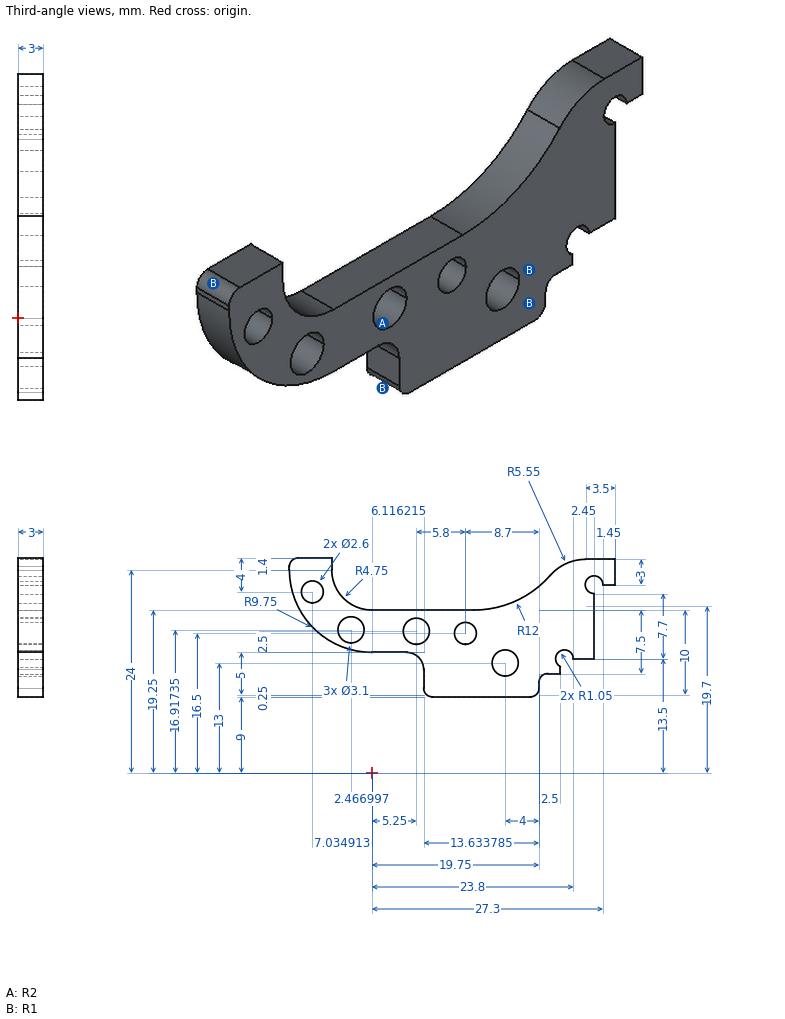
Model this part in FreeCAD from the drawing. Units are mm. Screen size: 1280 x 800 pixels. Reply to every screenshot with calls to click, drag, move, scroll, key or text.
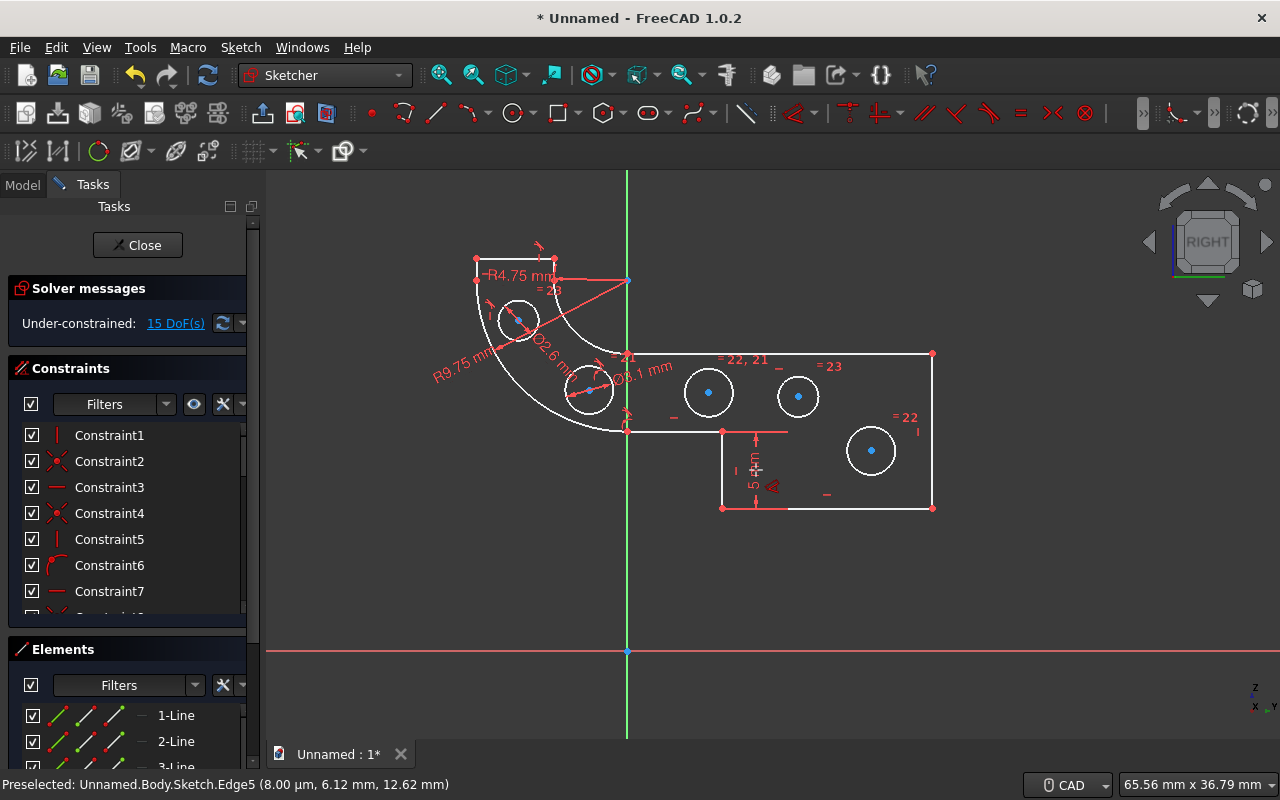
click(932, 462)
click(966, 431)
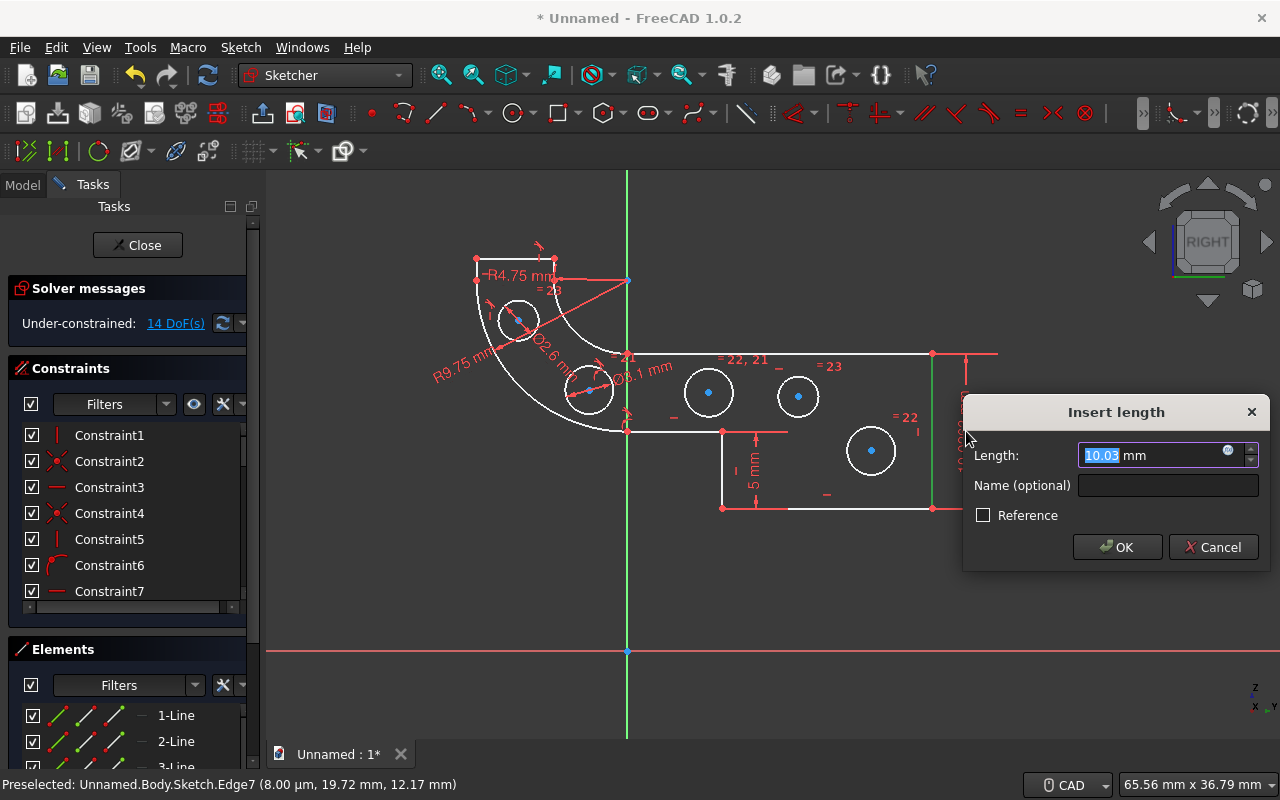
text(10)
key(Return)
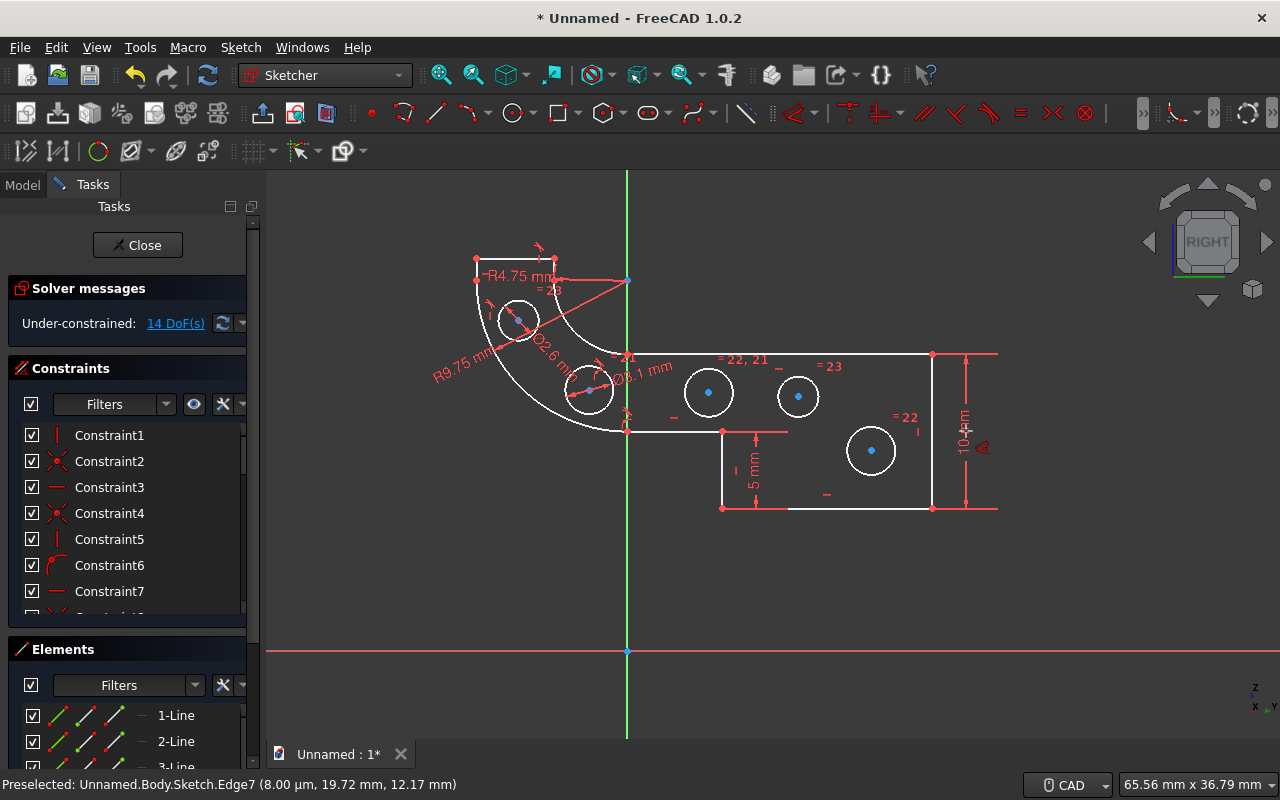
click(871, 451)
click(905, 551)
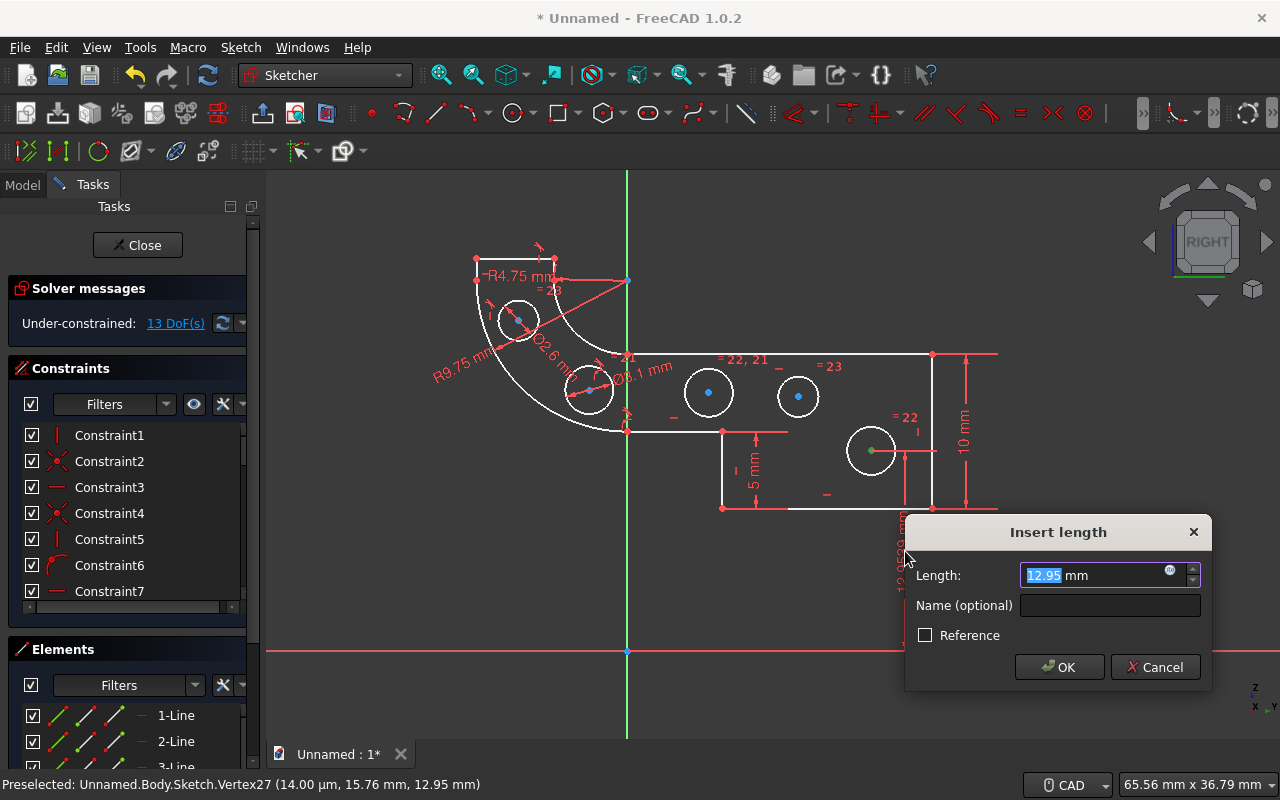
text(13)
key(Return)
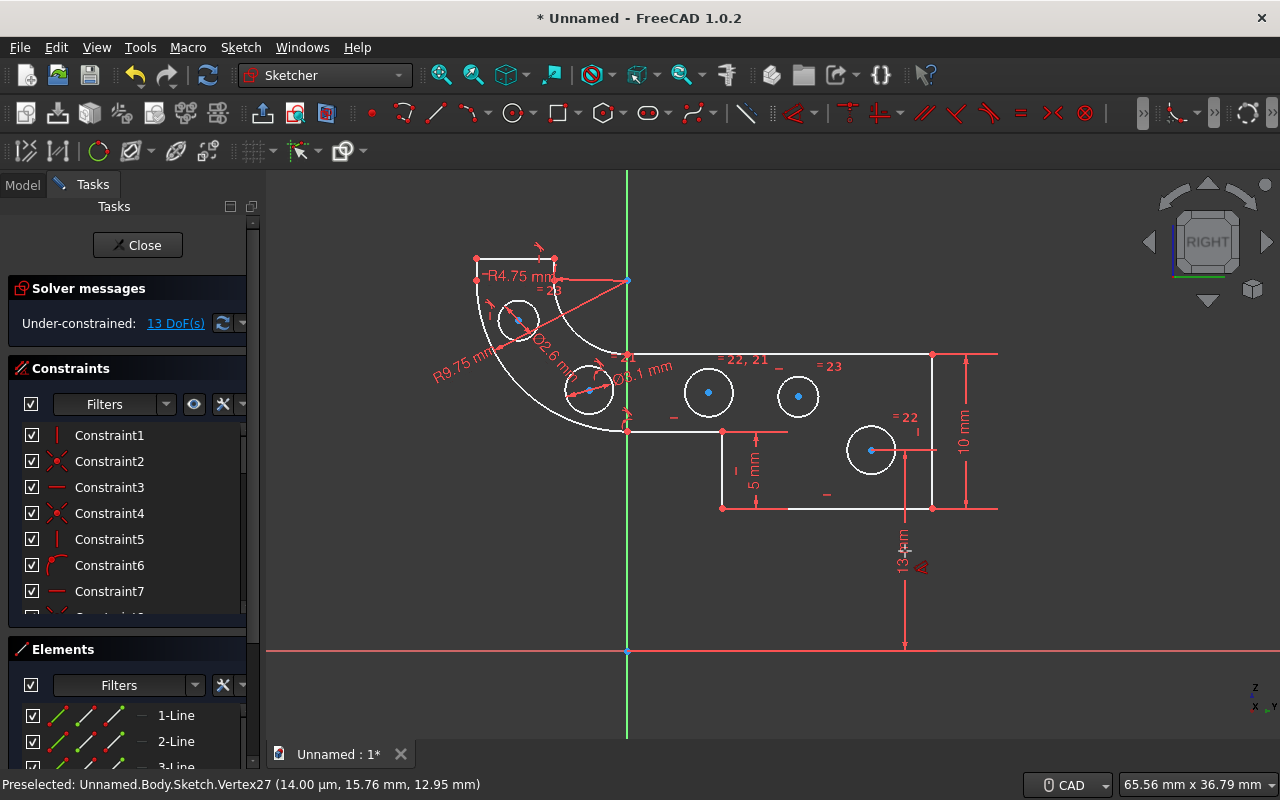
click(554, 259)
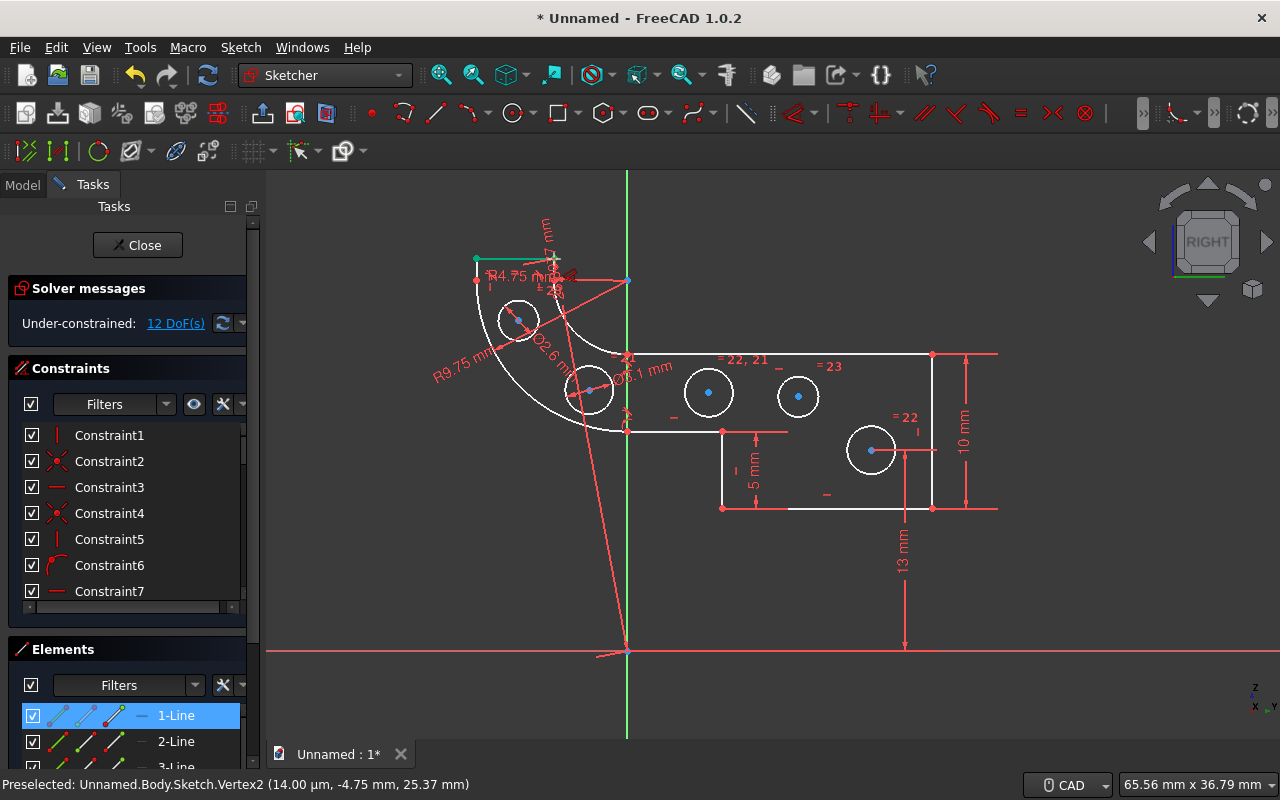
click(519, 321)
click(588, 304)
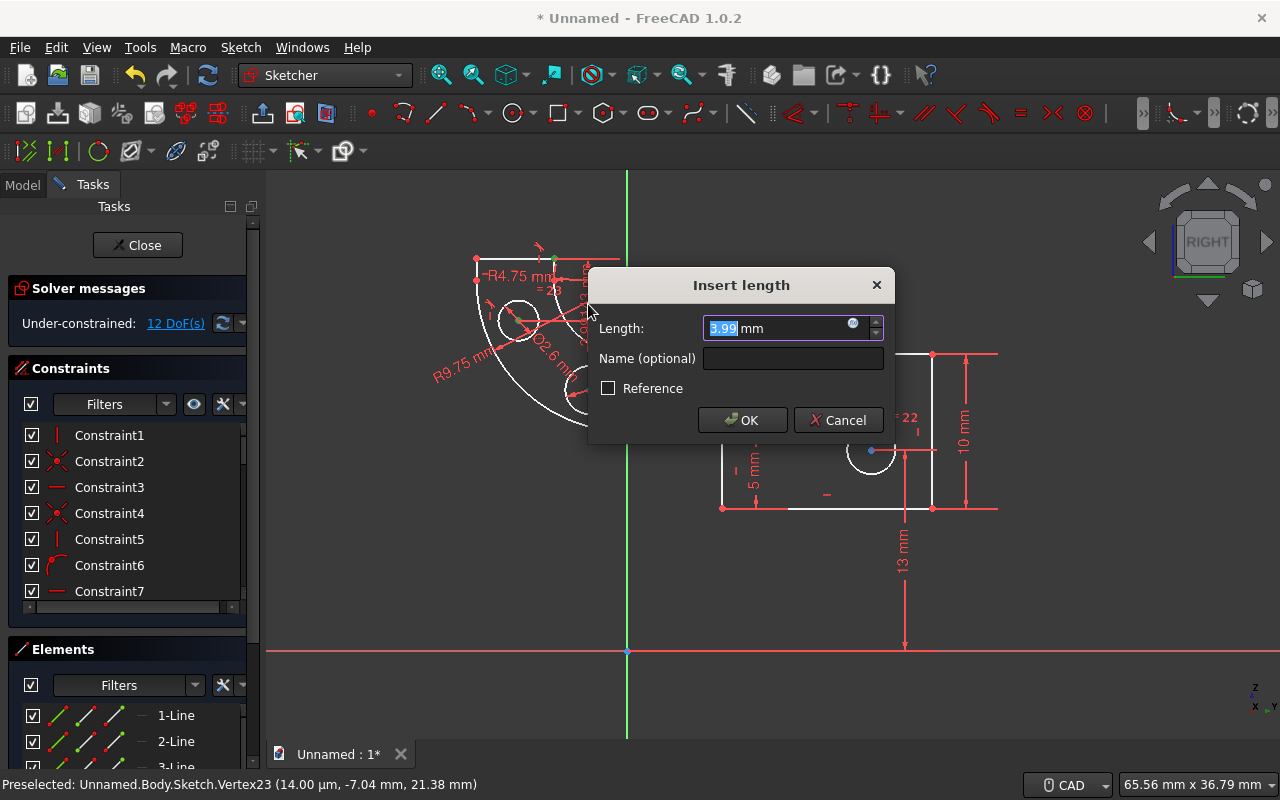
text(4)
key(Return)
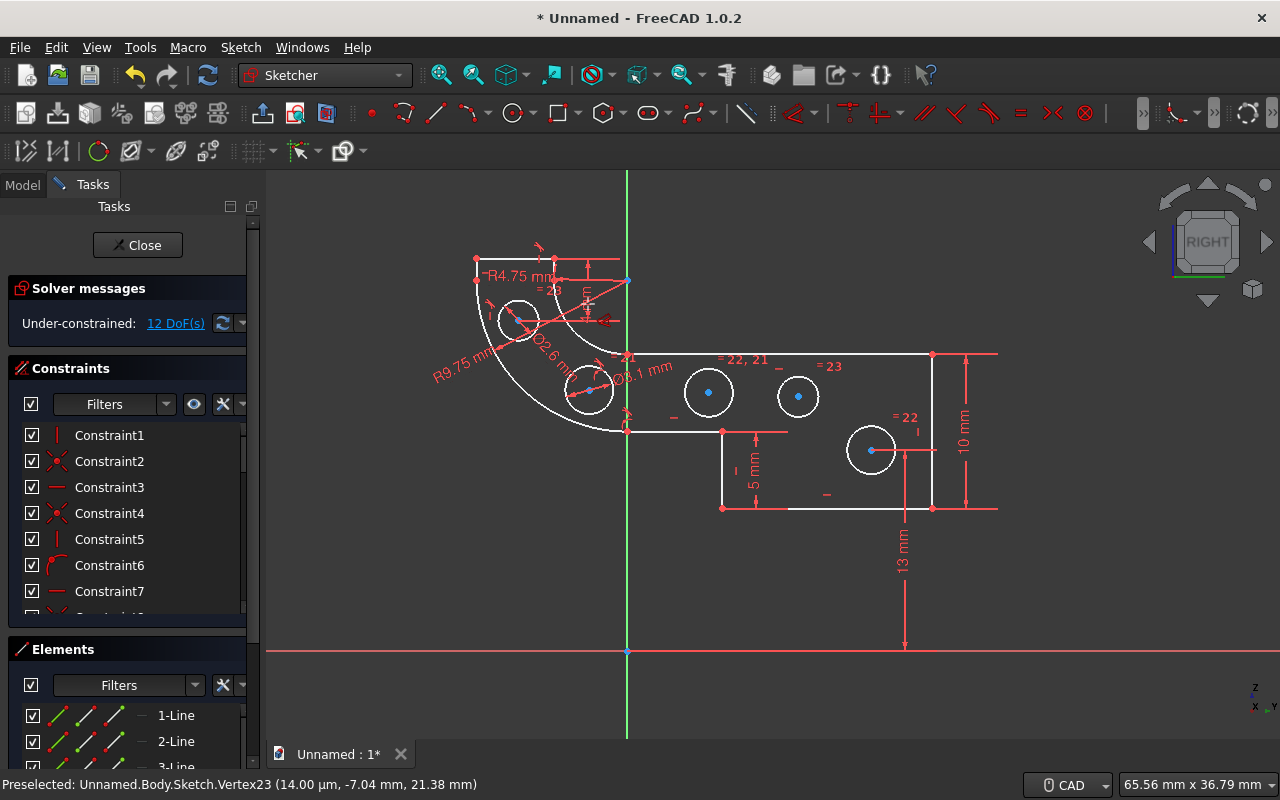
click(932, 509)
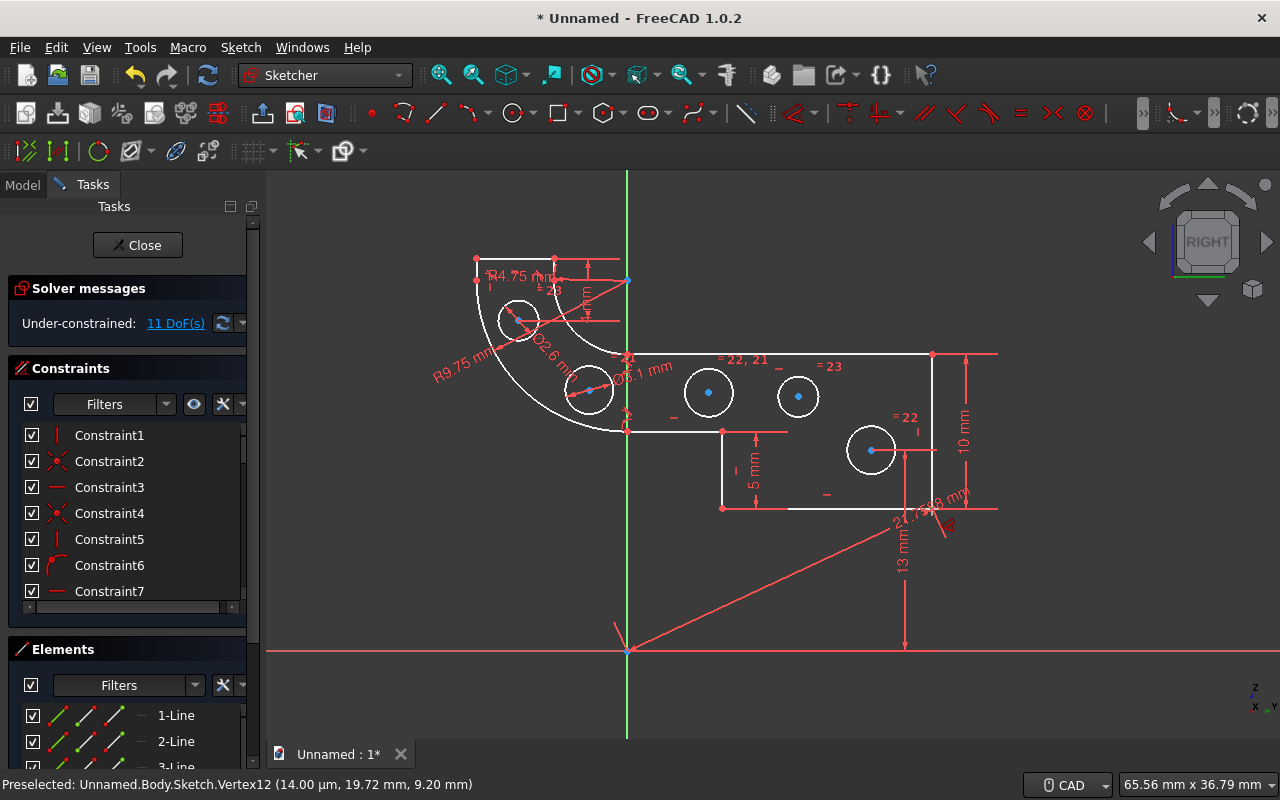
click(871, 450)
click(888, 416)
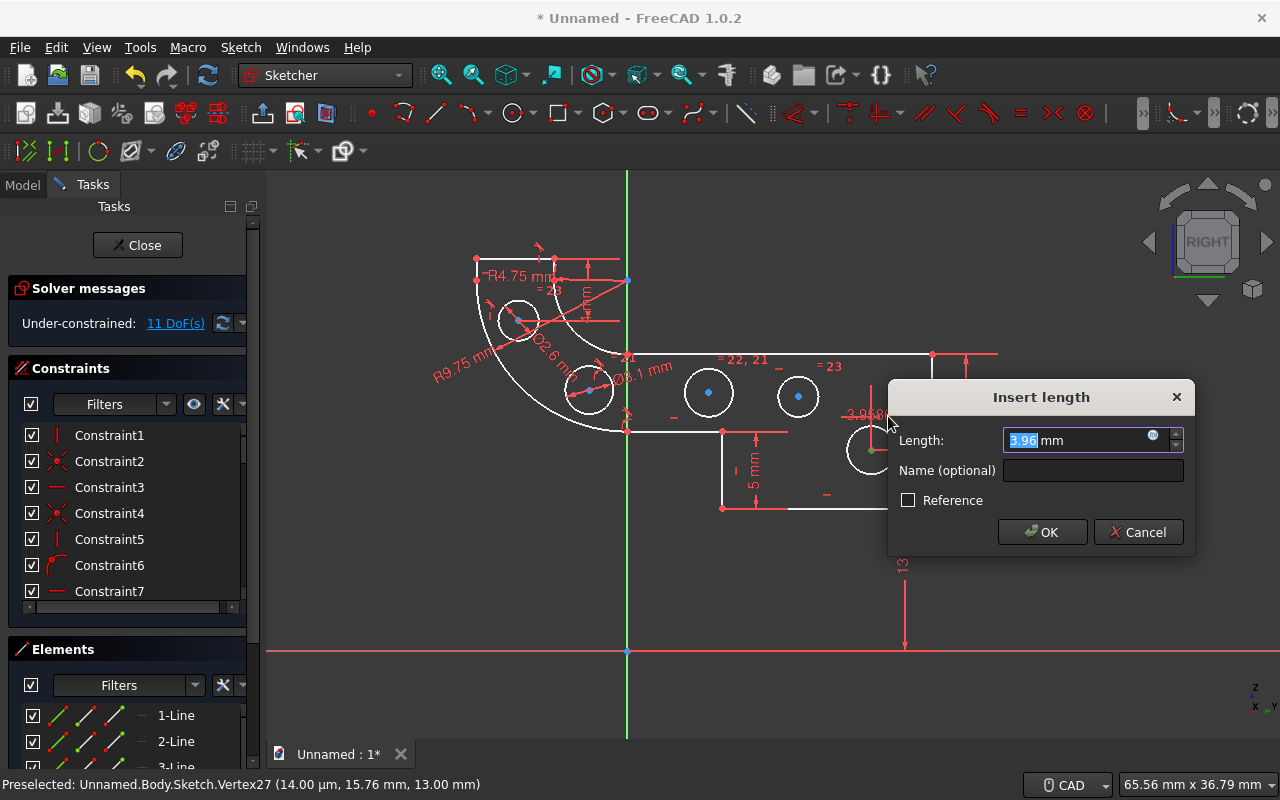
text(4)
key(Return)